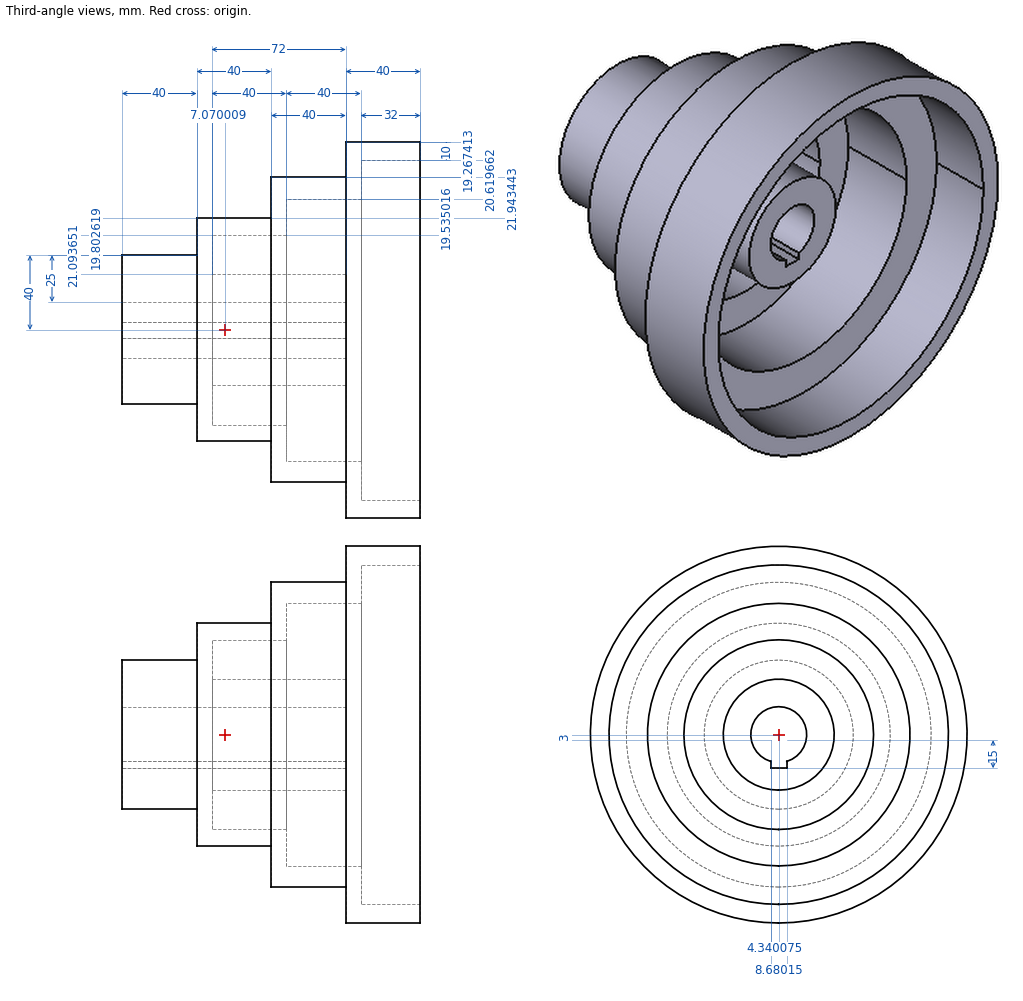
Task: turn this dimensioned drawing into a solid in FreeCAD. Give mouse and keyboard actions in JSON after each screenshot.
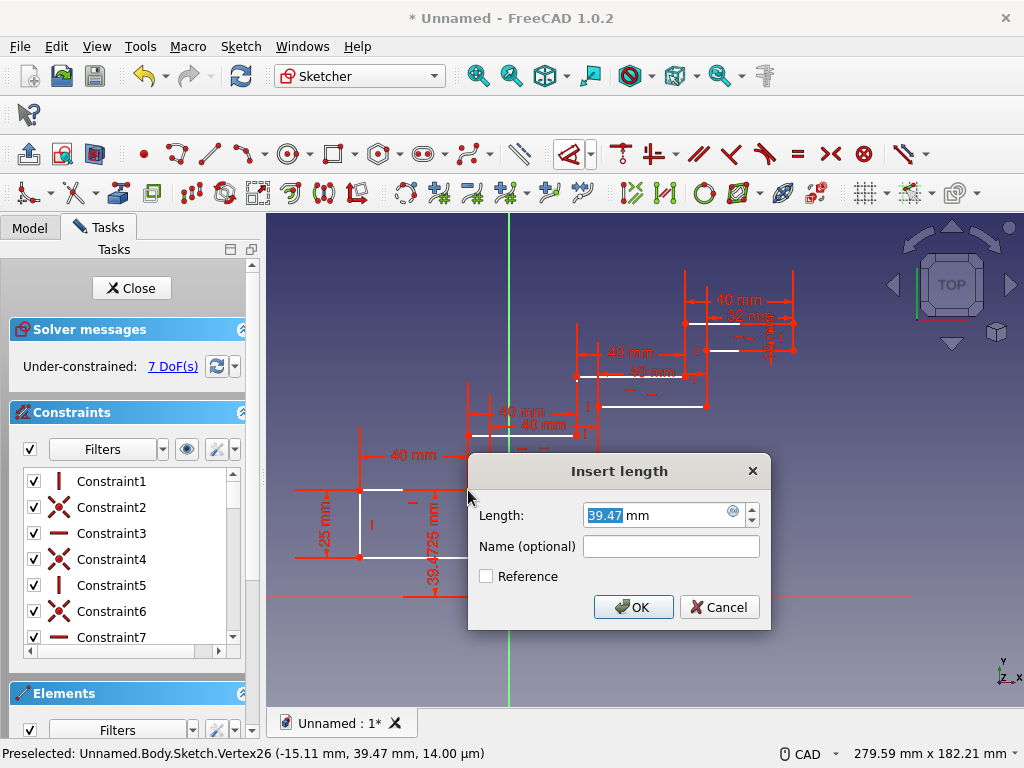
{"action": "type", "text": "40"}
{"action": "key", "text": "Return"}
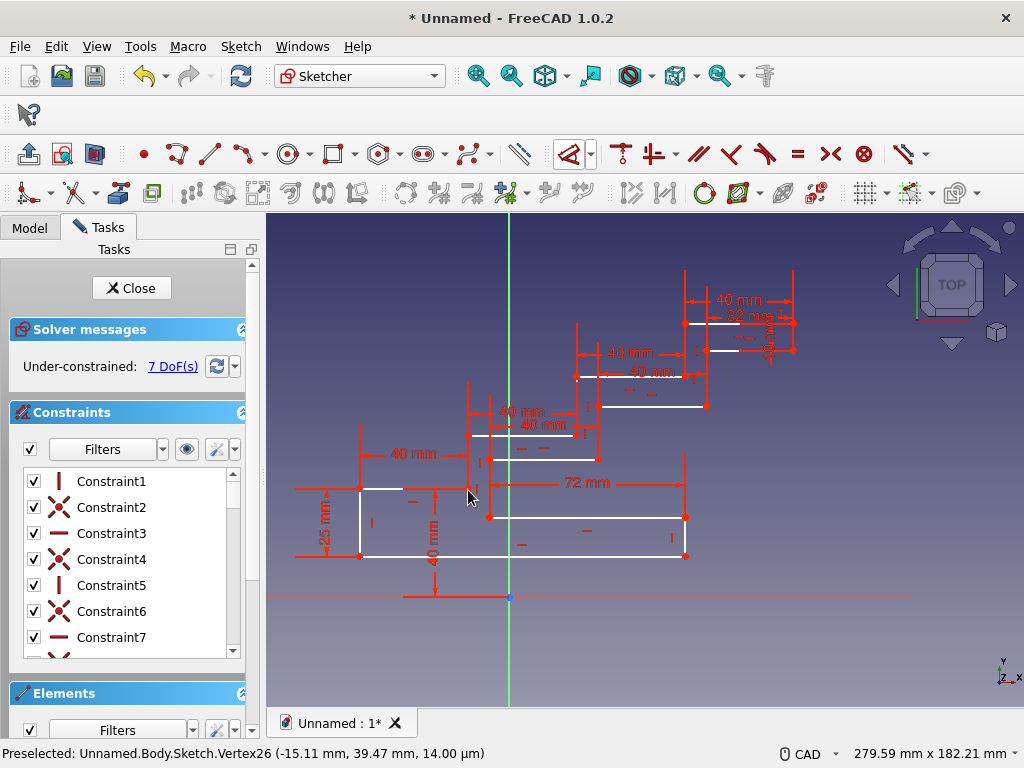
{"action": "left_click", "coordinate": [490, 501]}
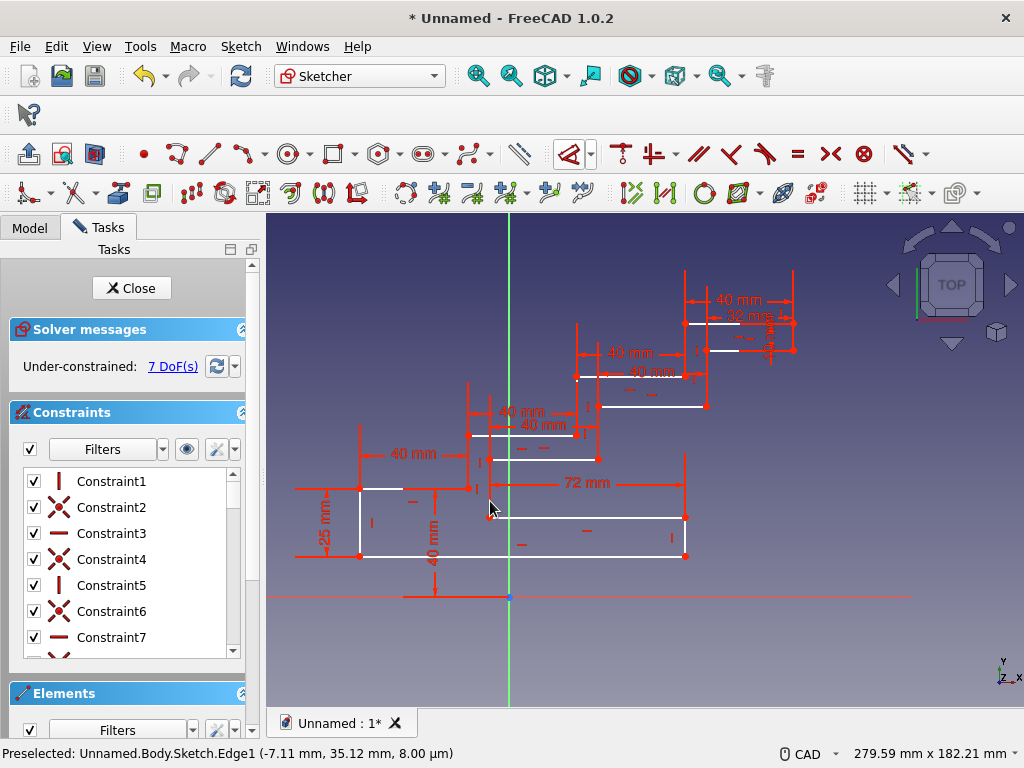
{"action": "left_click", "coordinate": [590, 154]}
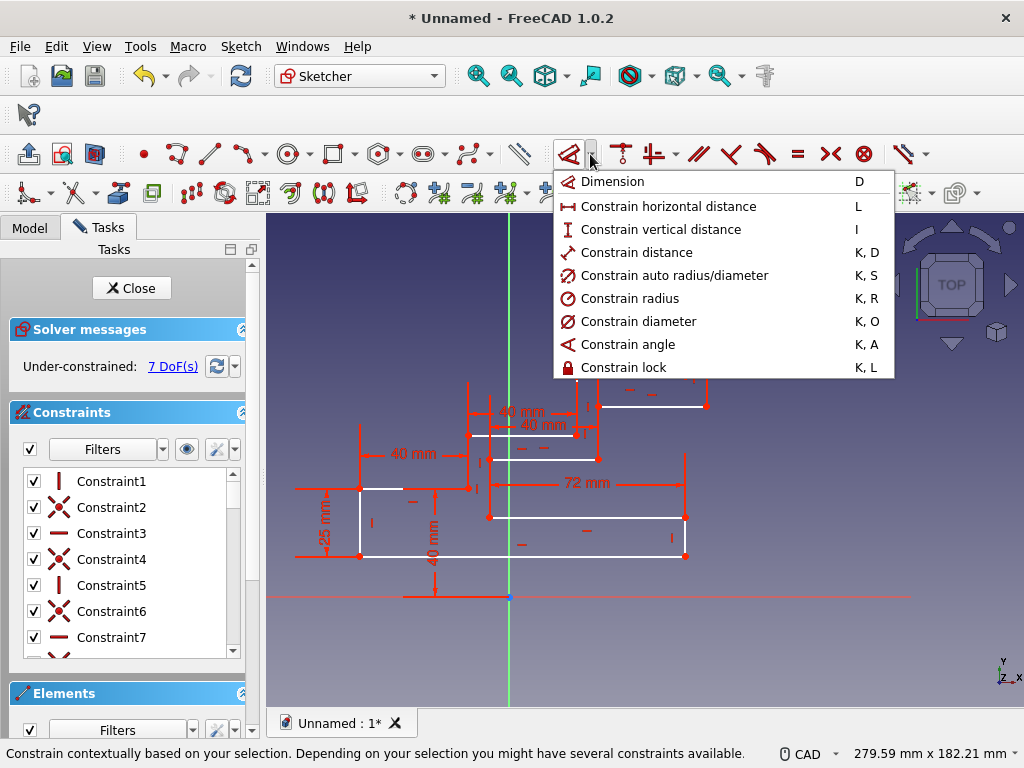
{"action": "left_click", "coordinate": [724, 230]}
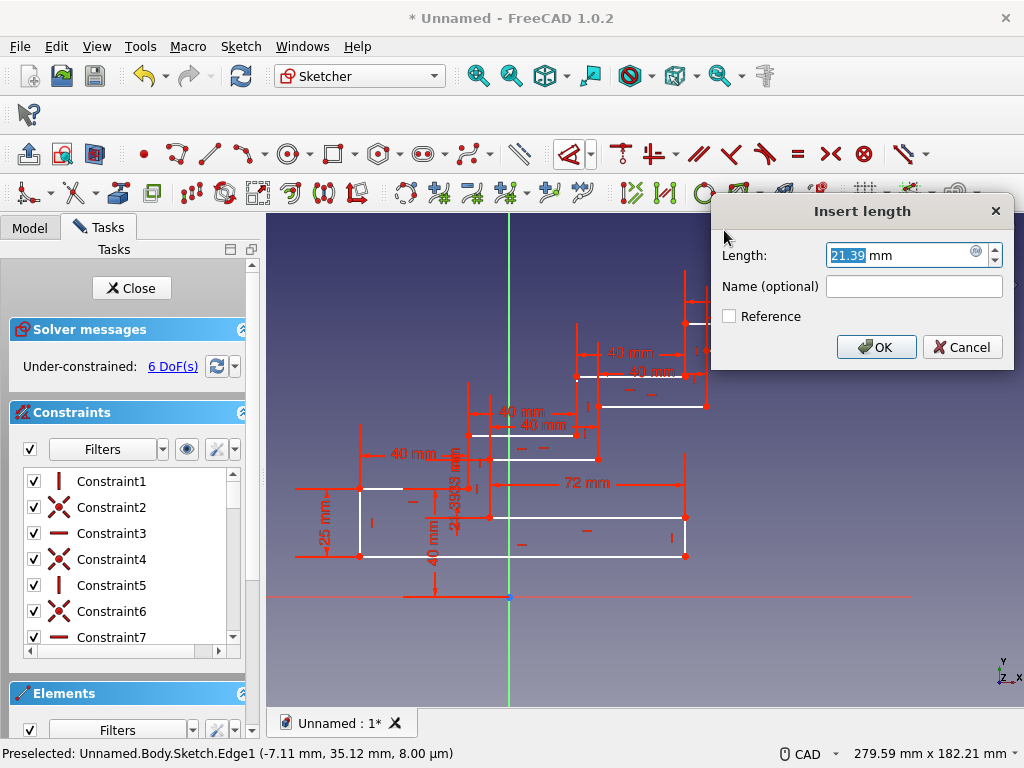
{"action": "type", "text": "21.093651"}
{"action": "key", "text": "Return"}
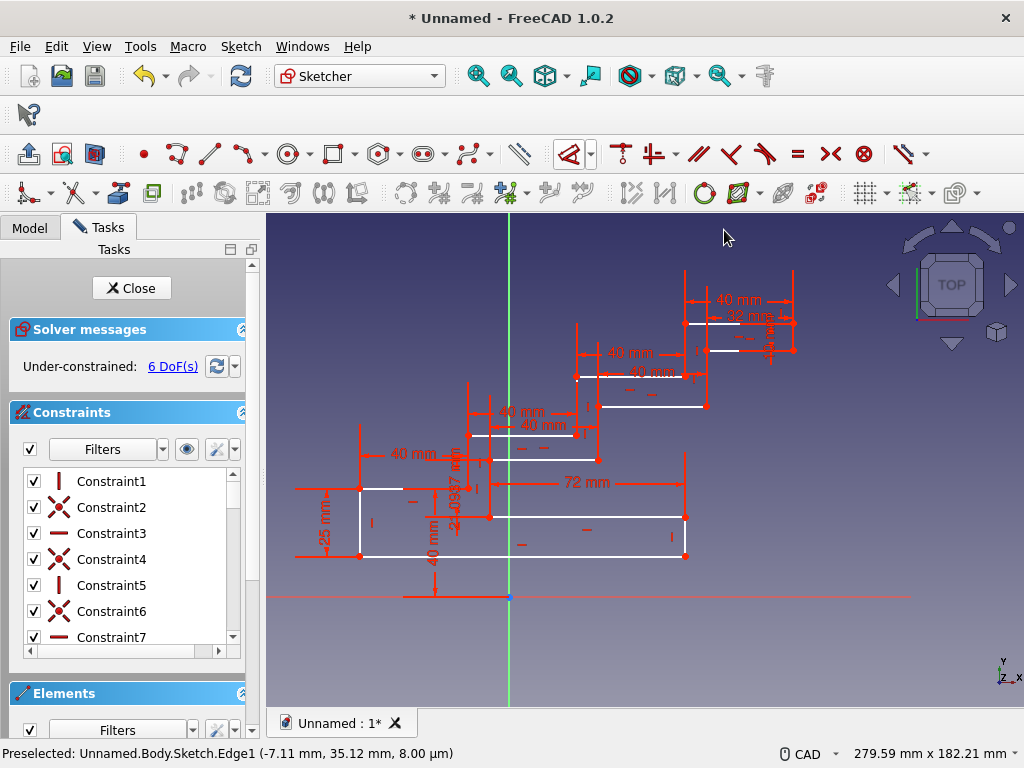
{"action": "left_click", "coordinate": [598, 444]}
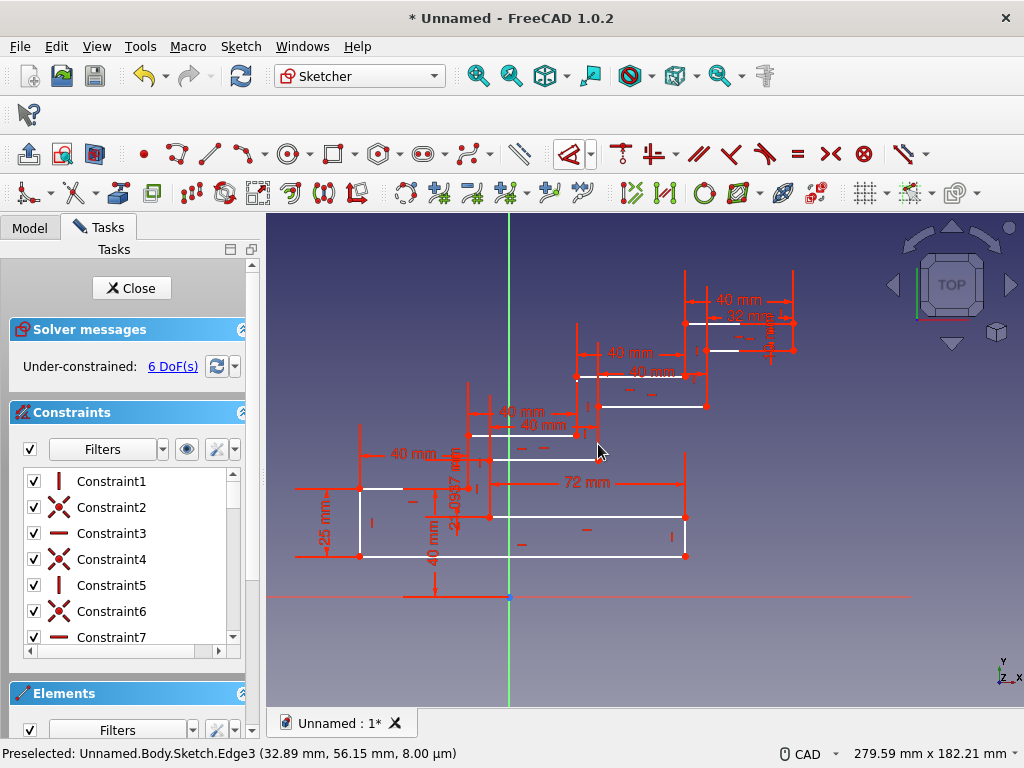
{"action": "left_click", "coordinate": [590, 154]}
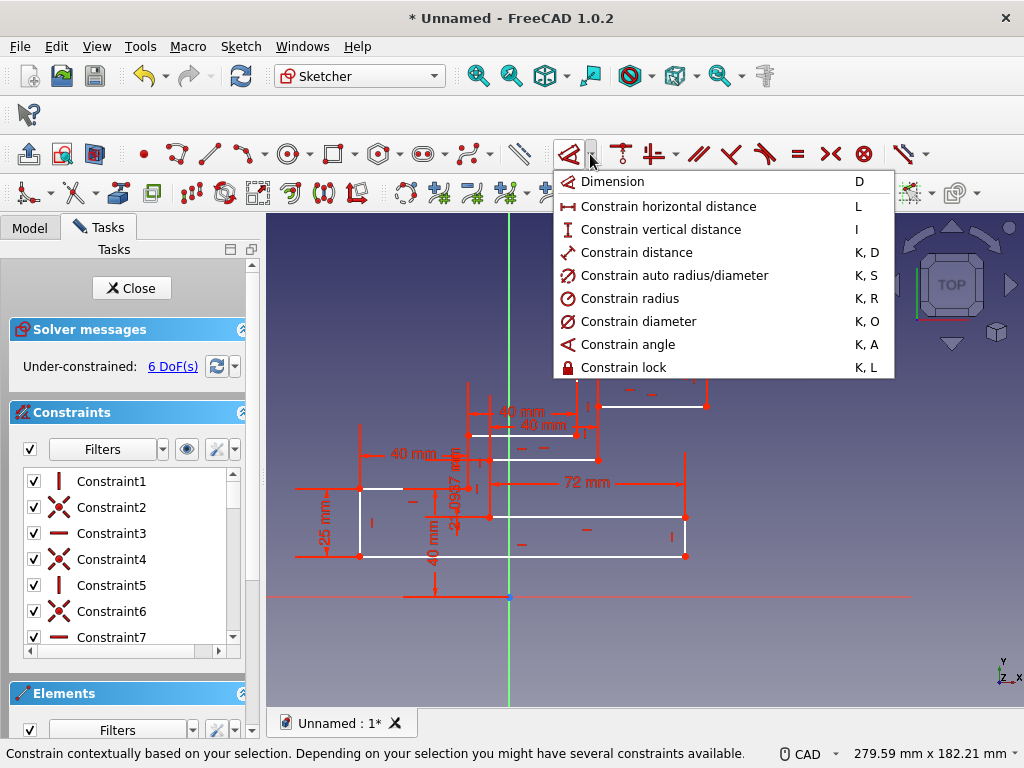
{"action": "left_click", "coordinate": [724, 230]}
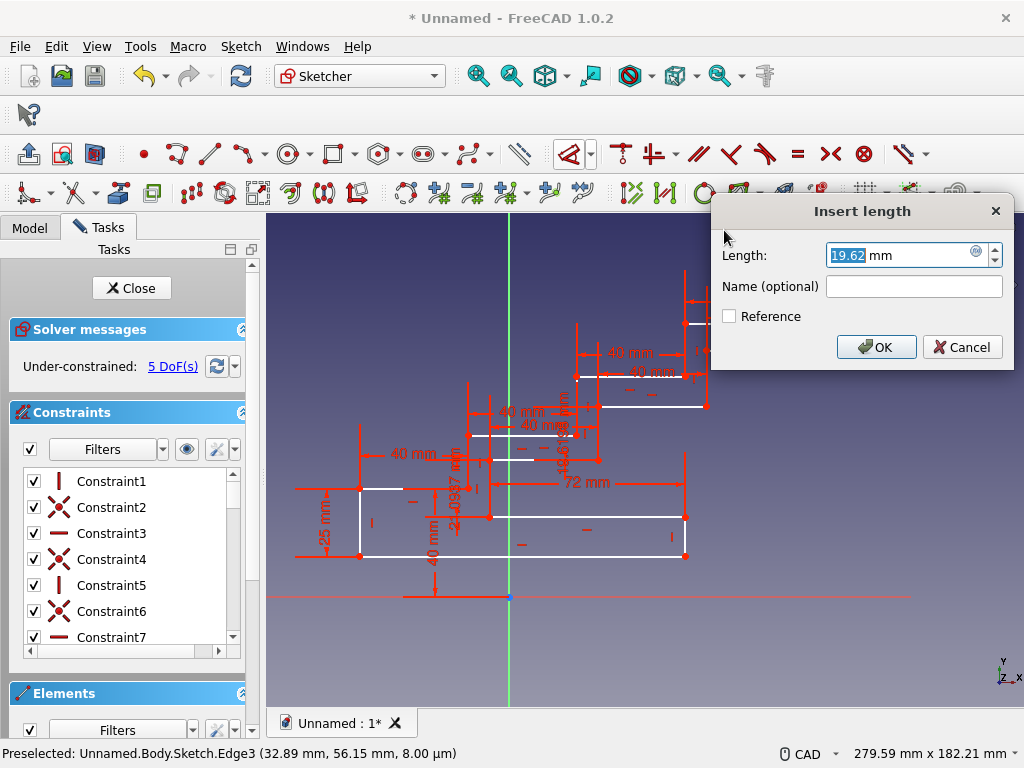
{"action": "type", "text": "19.535016"}
{"action": "key", "text": "Return"}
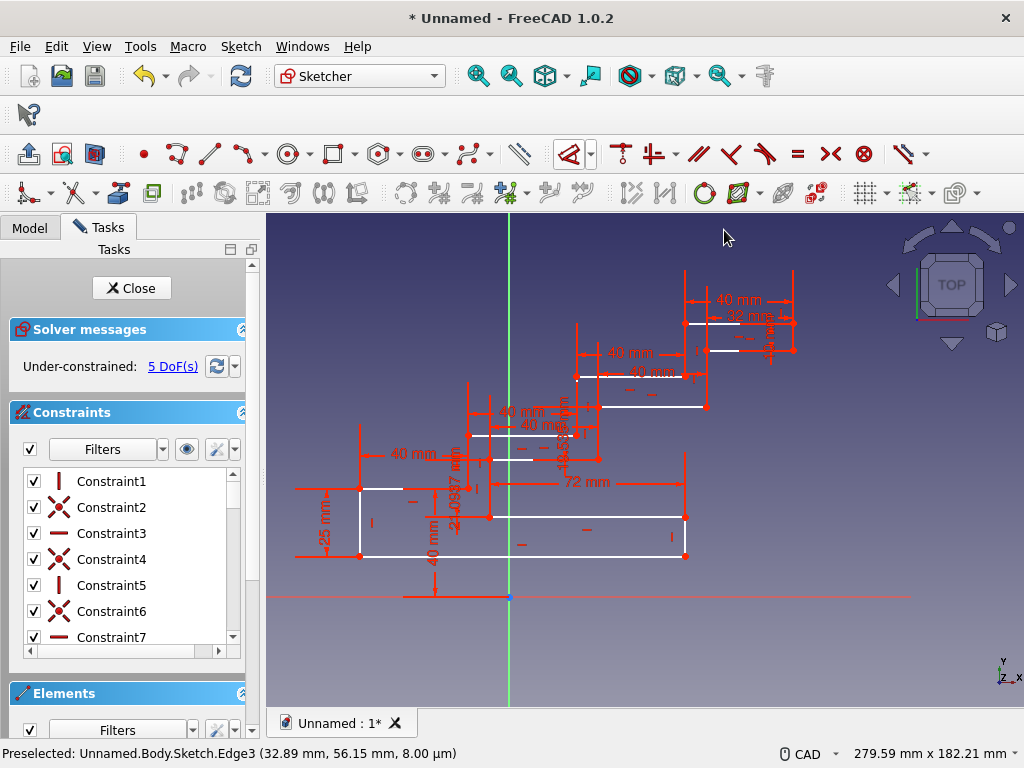
{"action": "left_click", "coordinate": [707, 390]}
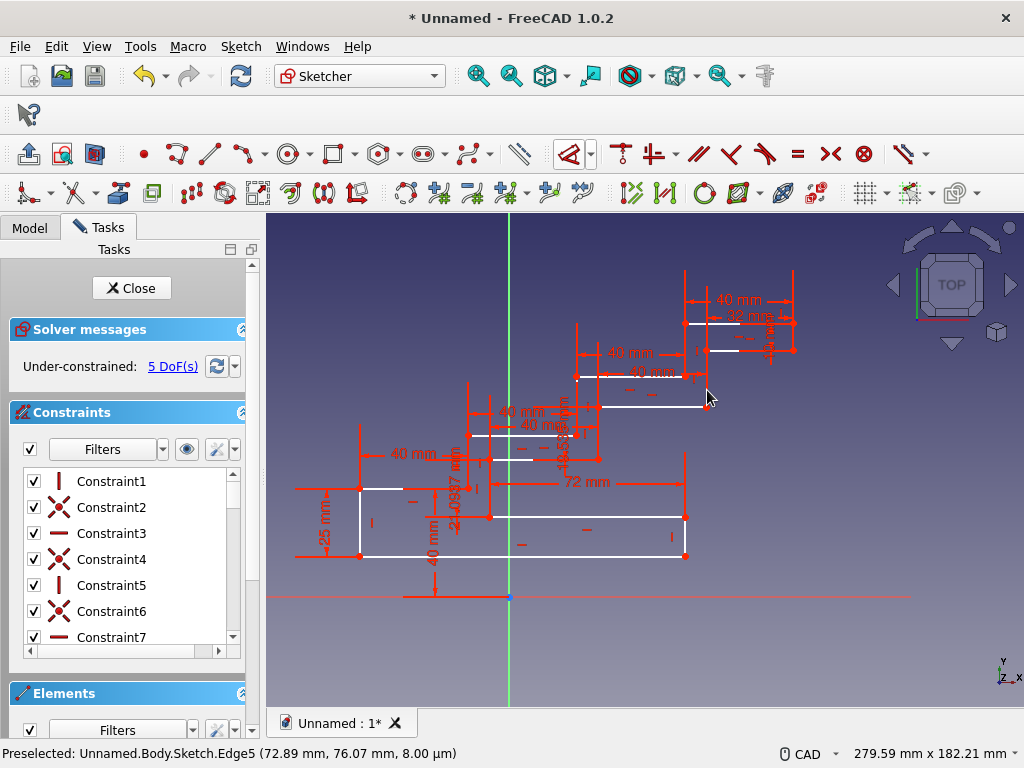
{"action": "left_click", "coordinate": [590, 154]}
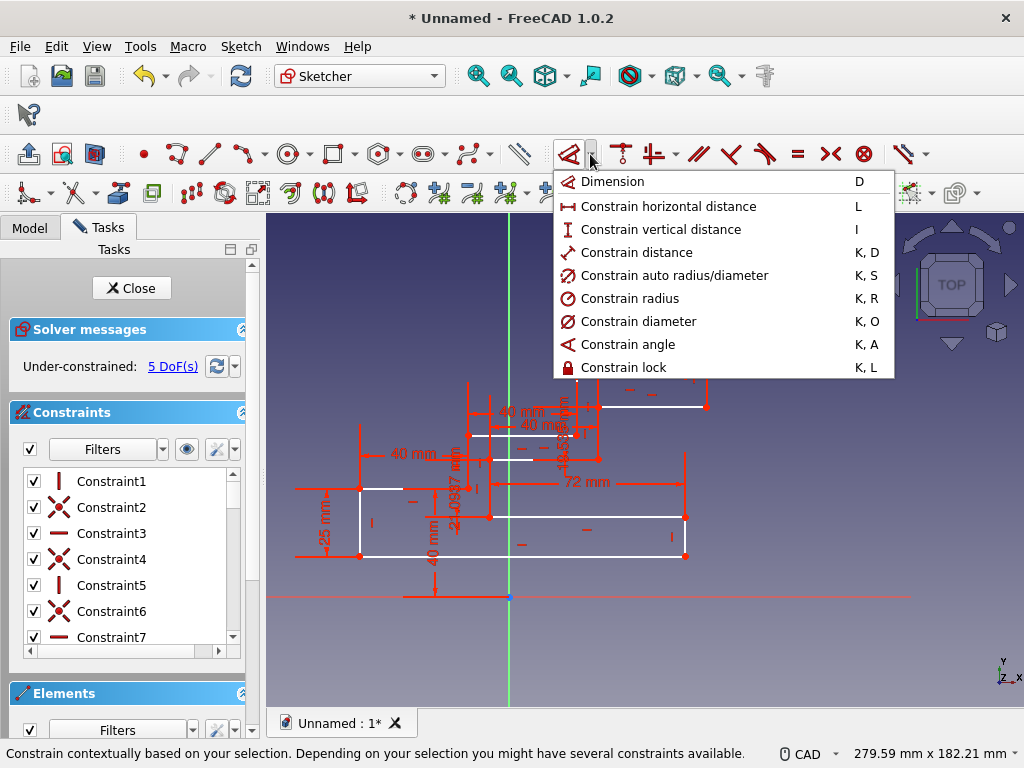
{"action": "left_click", "coordinate": [724, 230]}